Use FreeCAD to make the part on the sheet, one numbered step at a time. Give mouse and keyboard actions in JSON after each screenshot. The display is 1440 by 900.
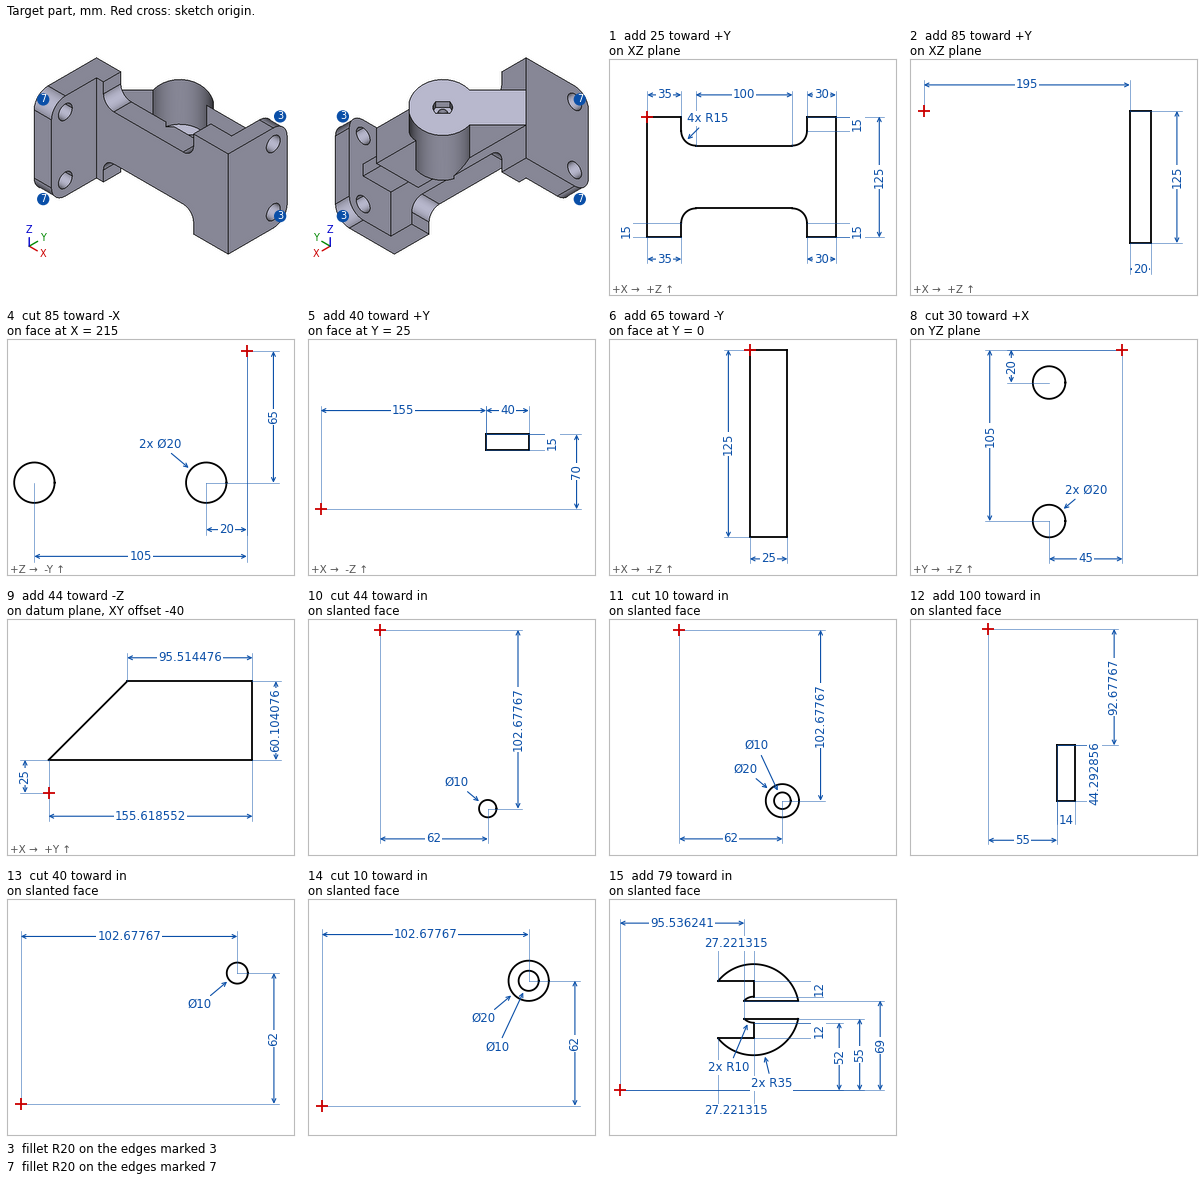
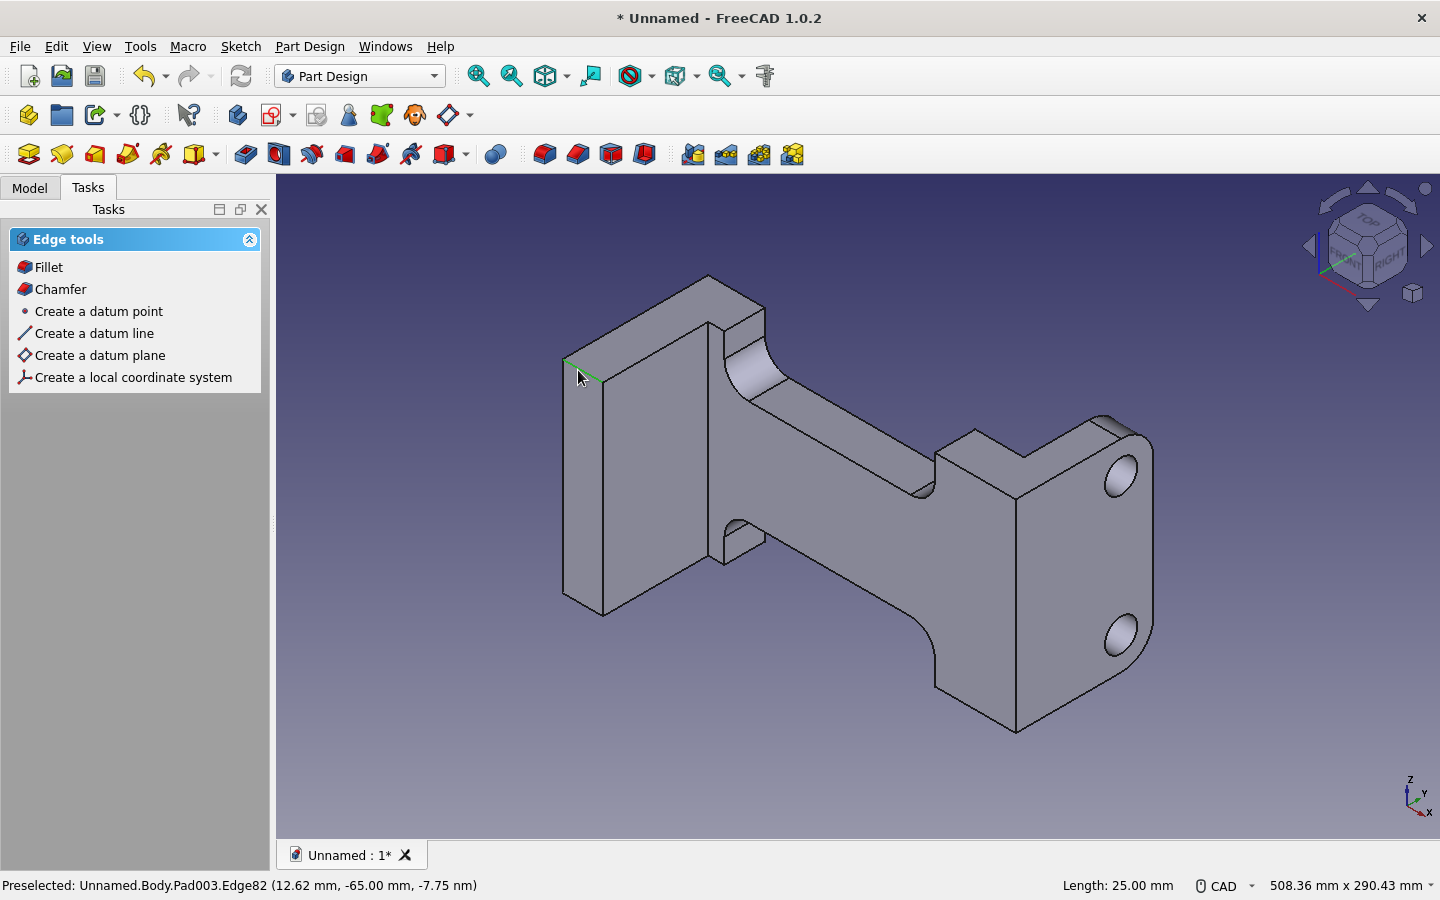
{"action": "key", "text": "1"}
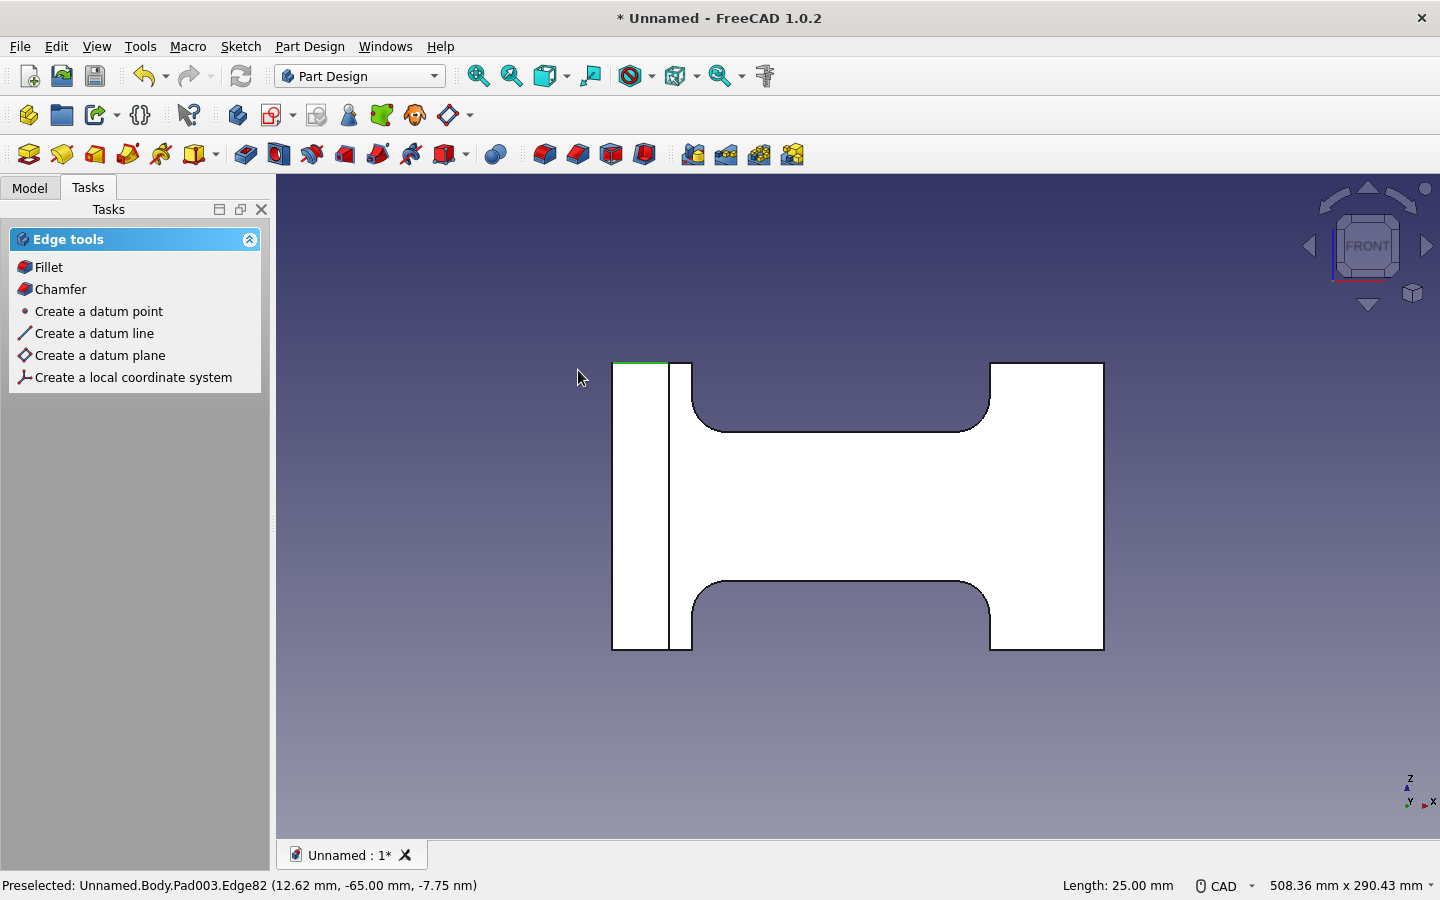
{"action": "key", "text": "v f"}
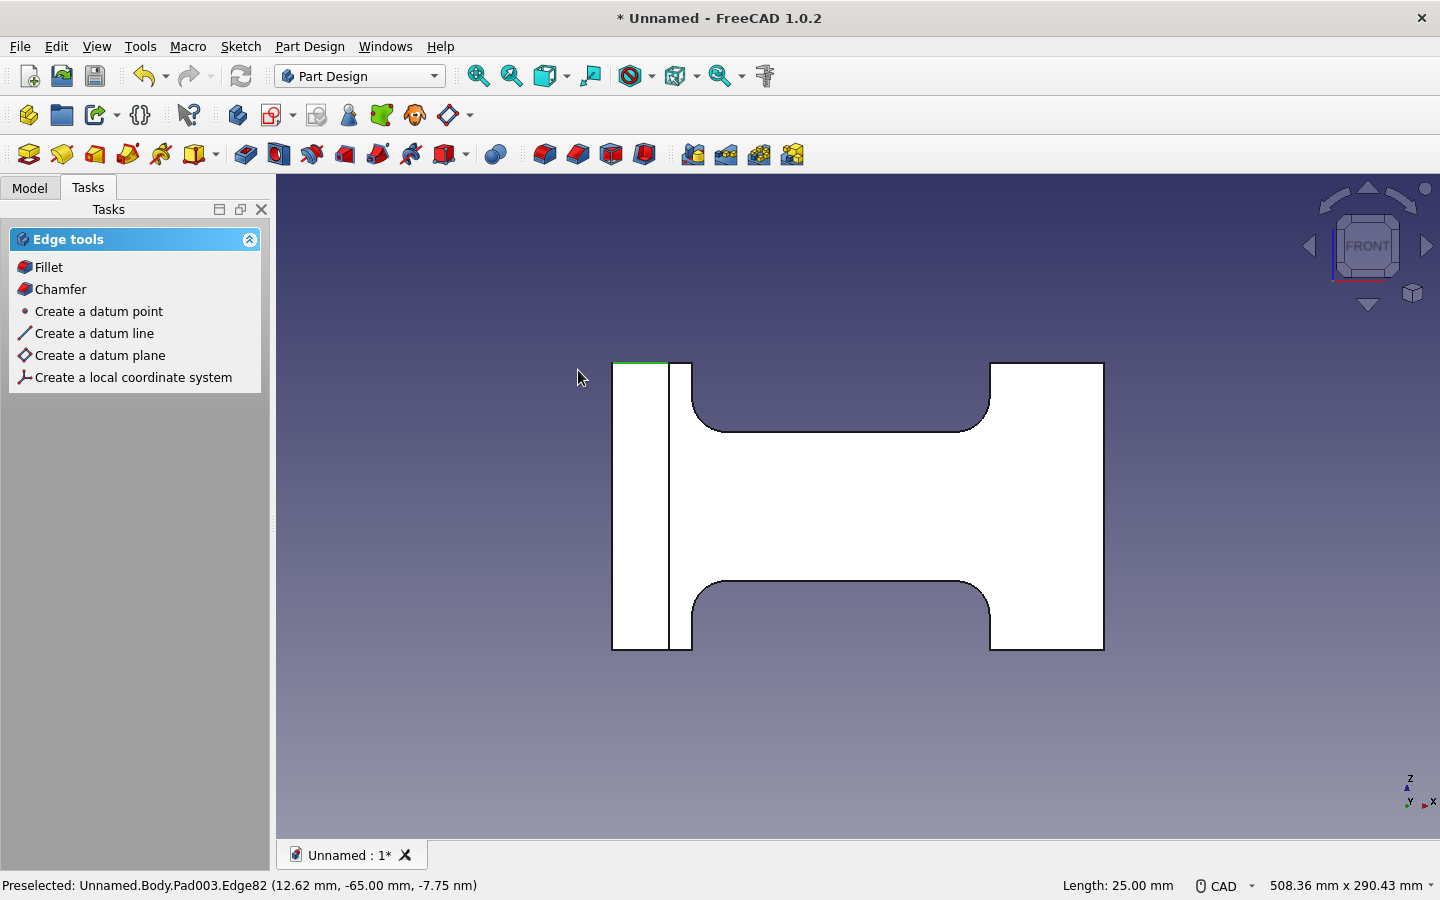
{"action": "key", "text": "3"}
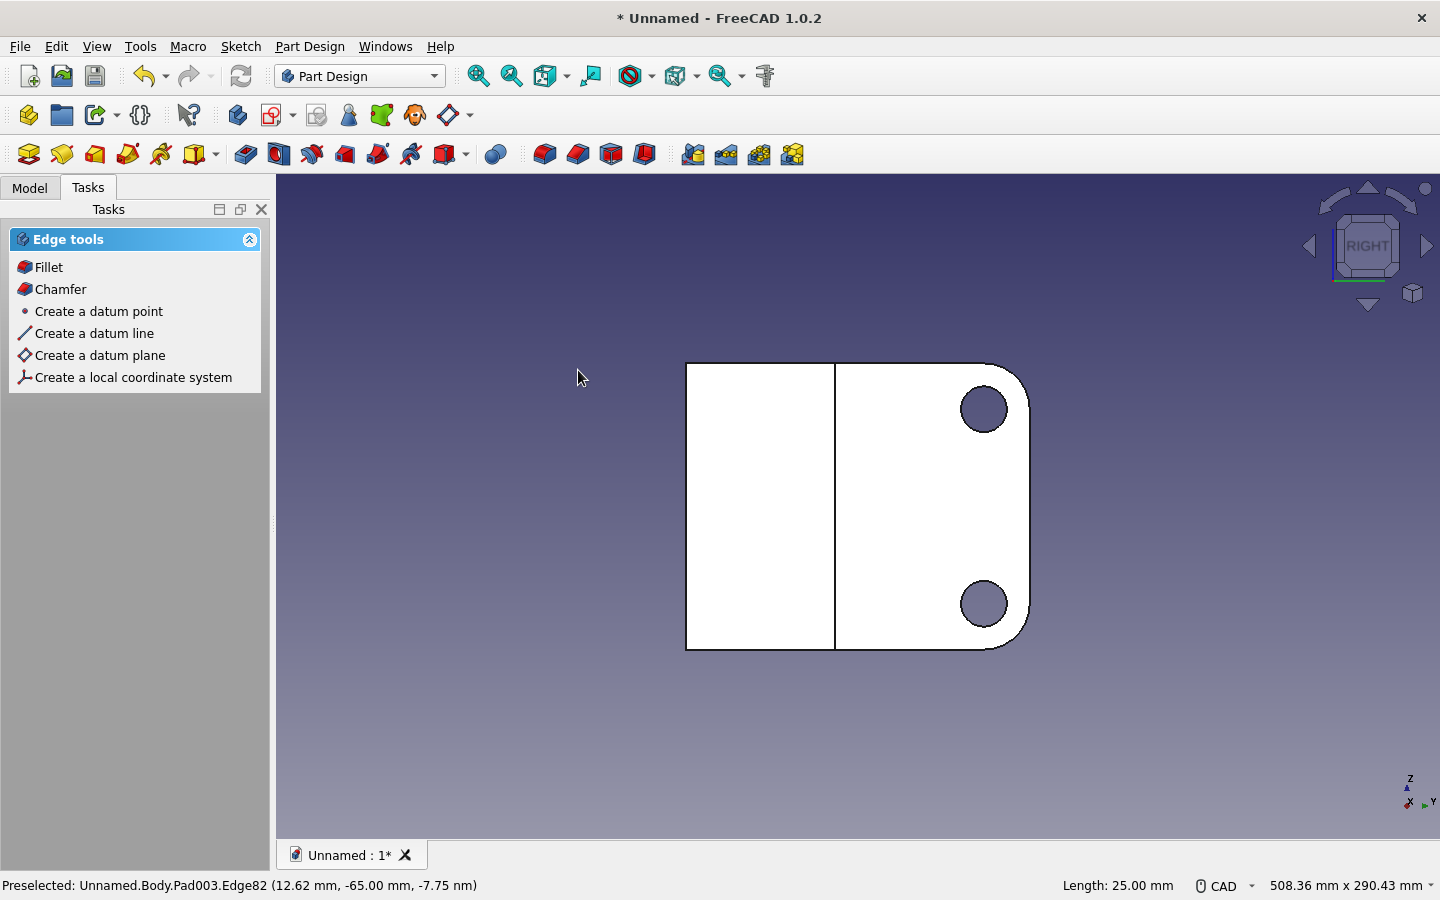
{"action": "left_click", "coordinate": [479, 76]}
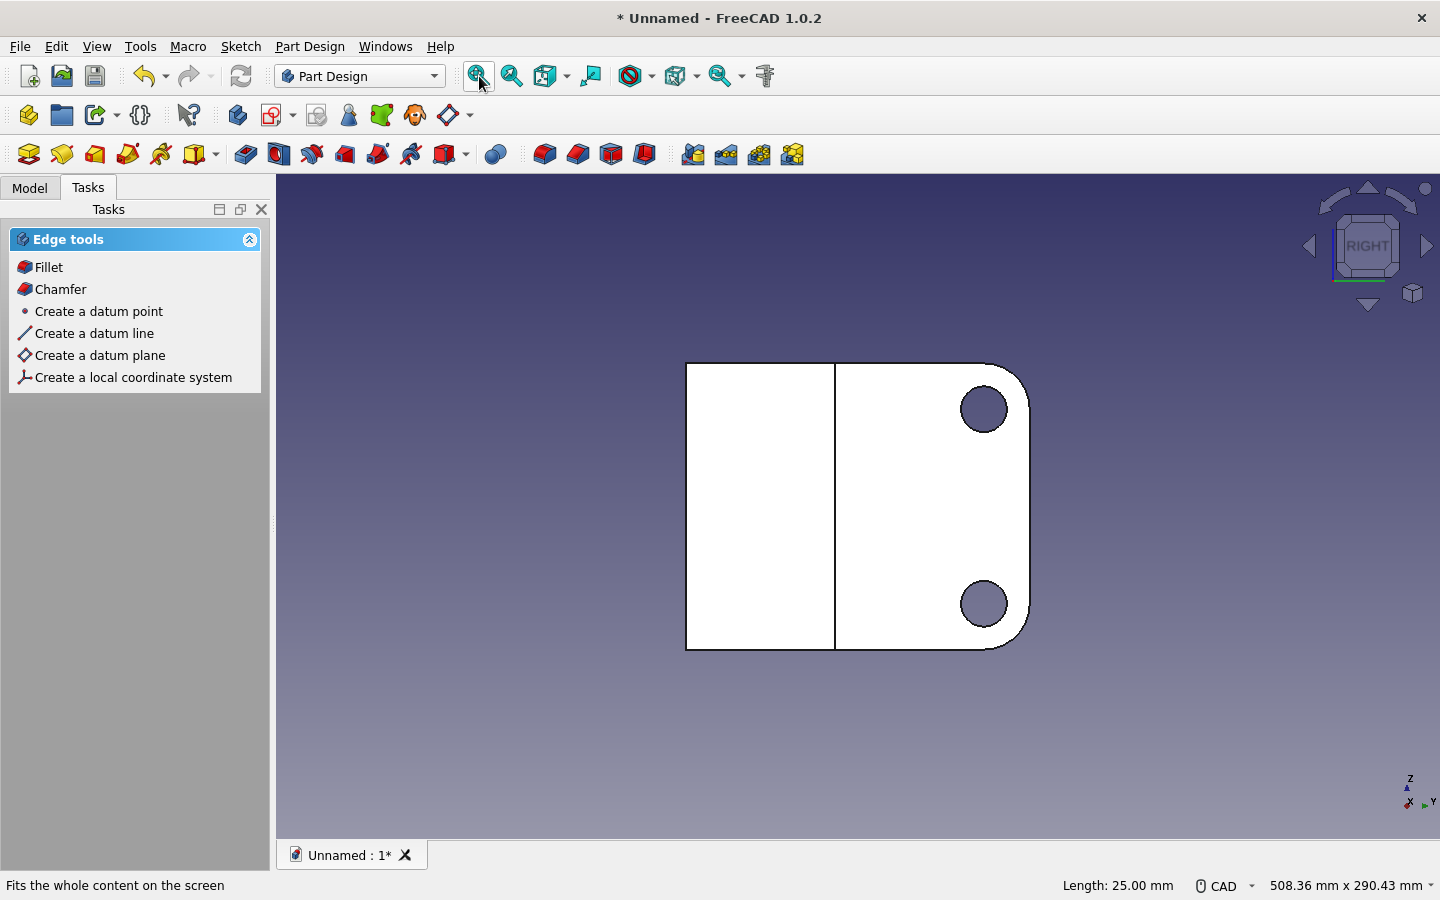
{"action": "key", "text": "5"}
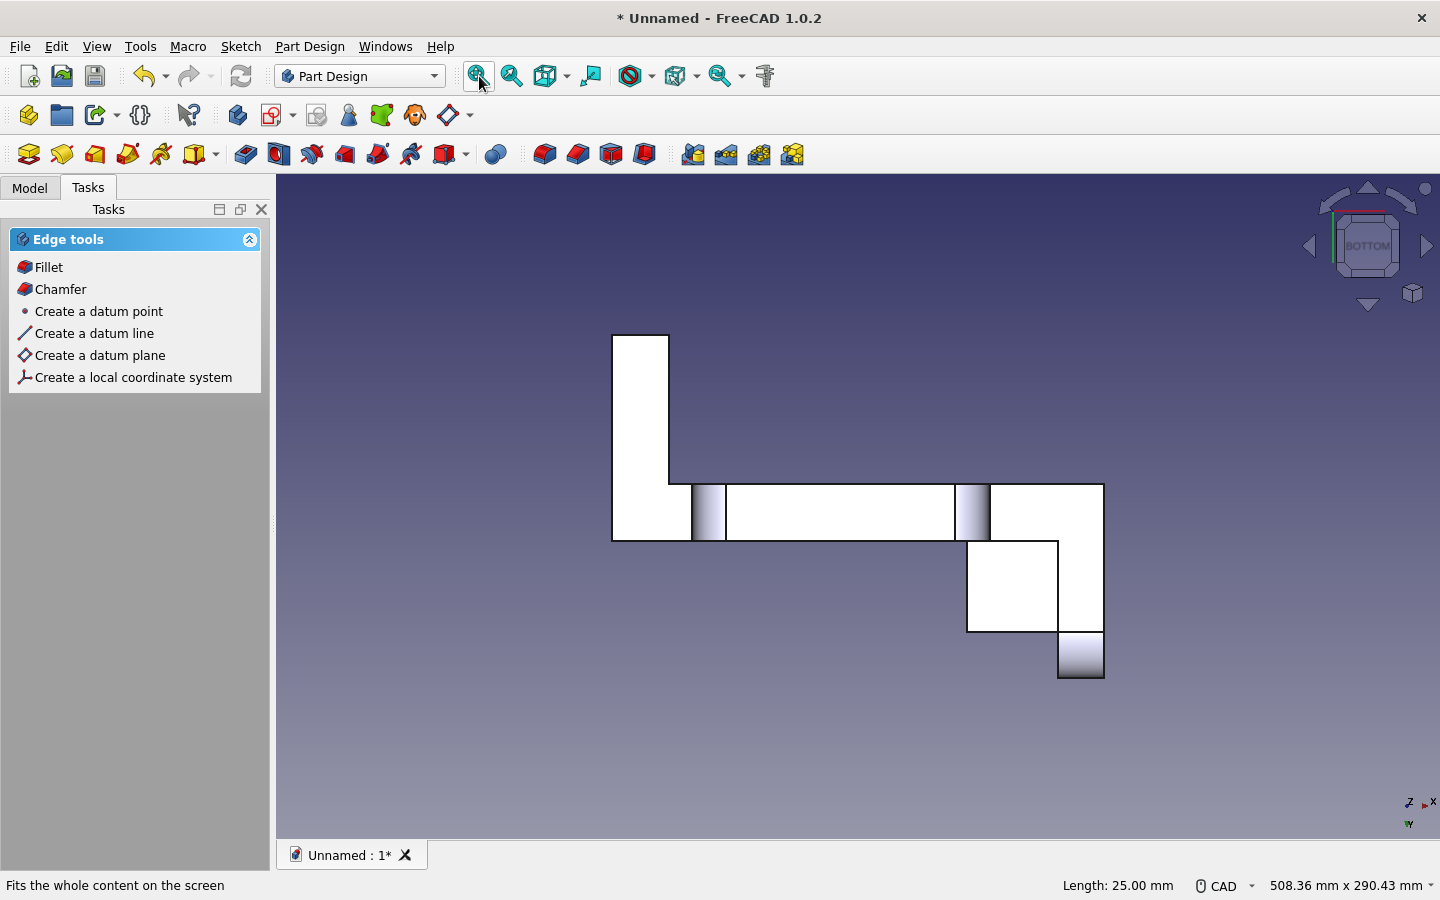
{"action": "left_click", "coordinate": [640, 334], "text": "ctrl"}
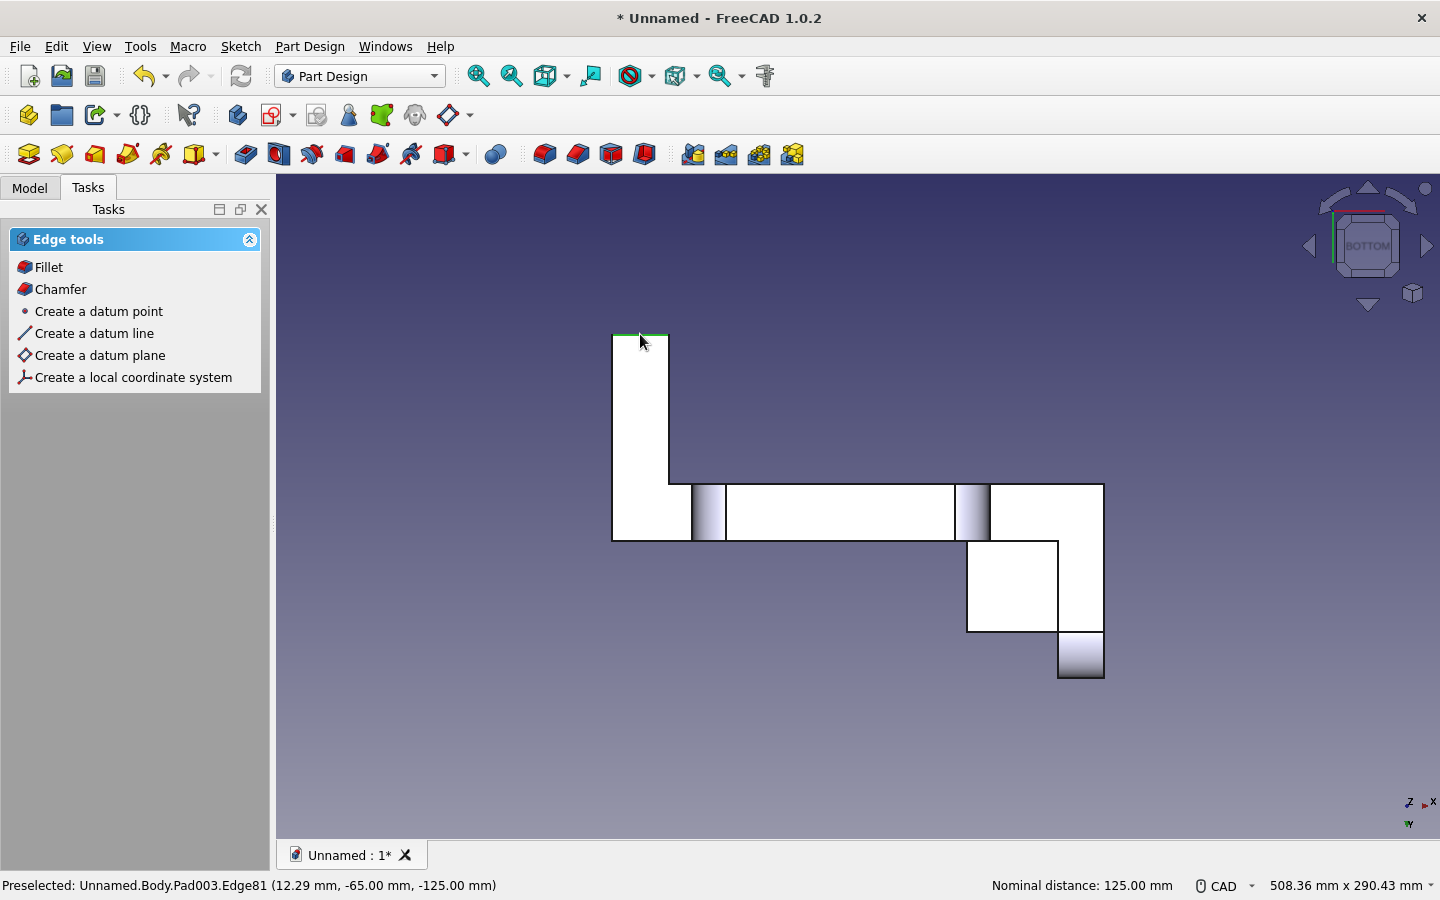
{"action": "left_click", "coordinate": [545, 154]}